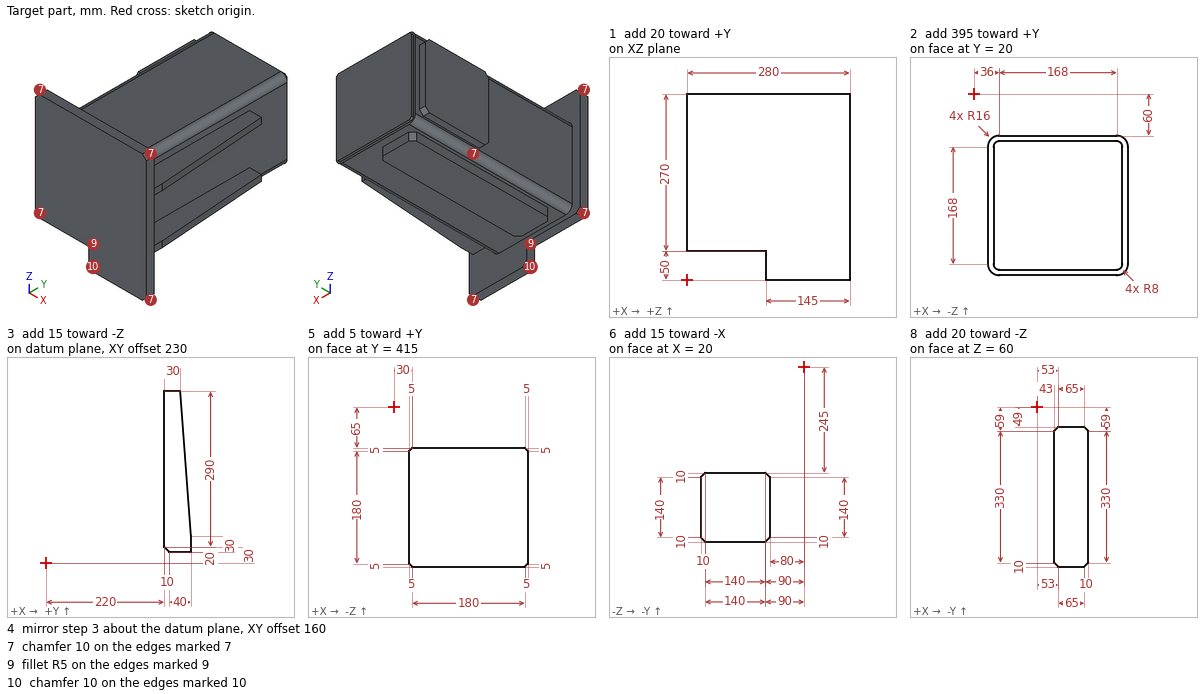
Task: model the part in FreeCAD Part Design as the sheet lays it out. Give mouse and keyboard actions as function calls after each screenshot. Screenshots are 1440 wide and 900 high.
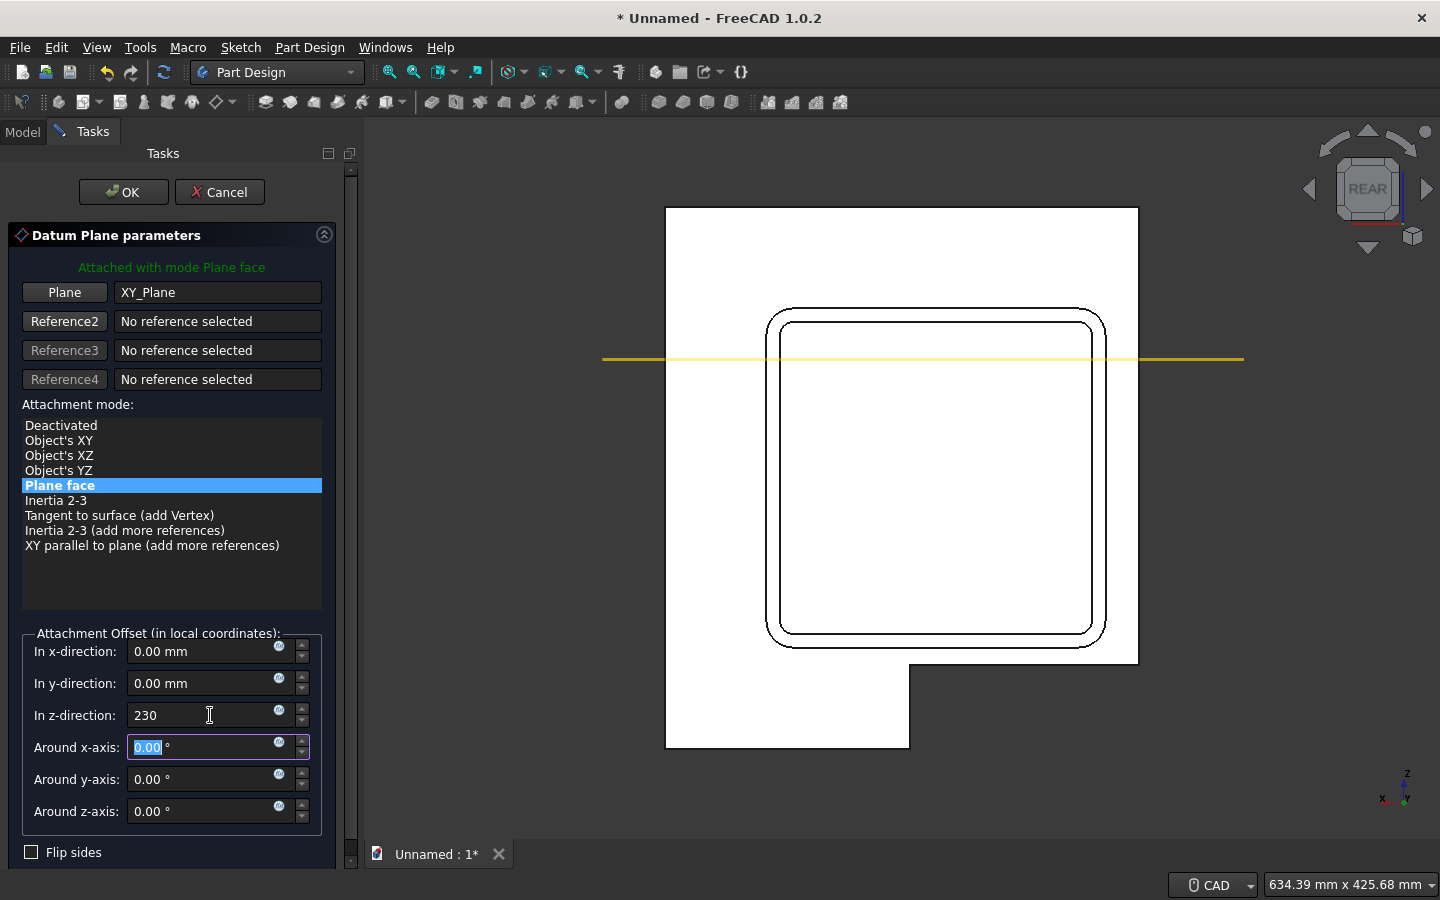
click(124, 192)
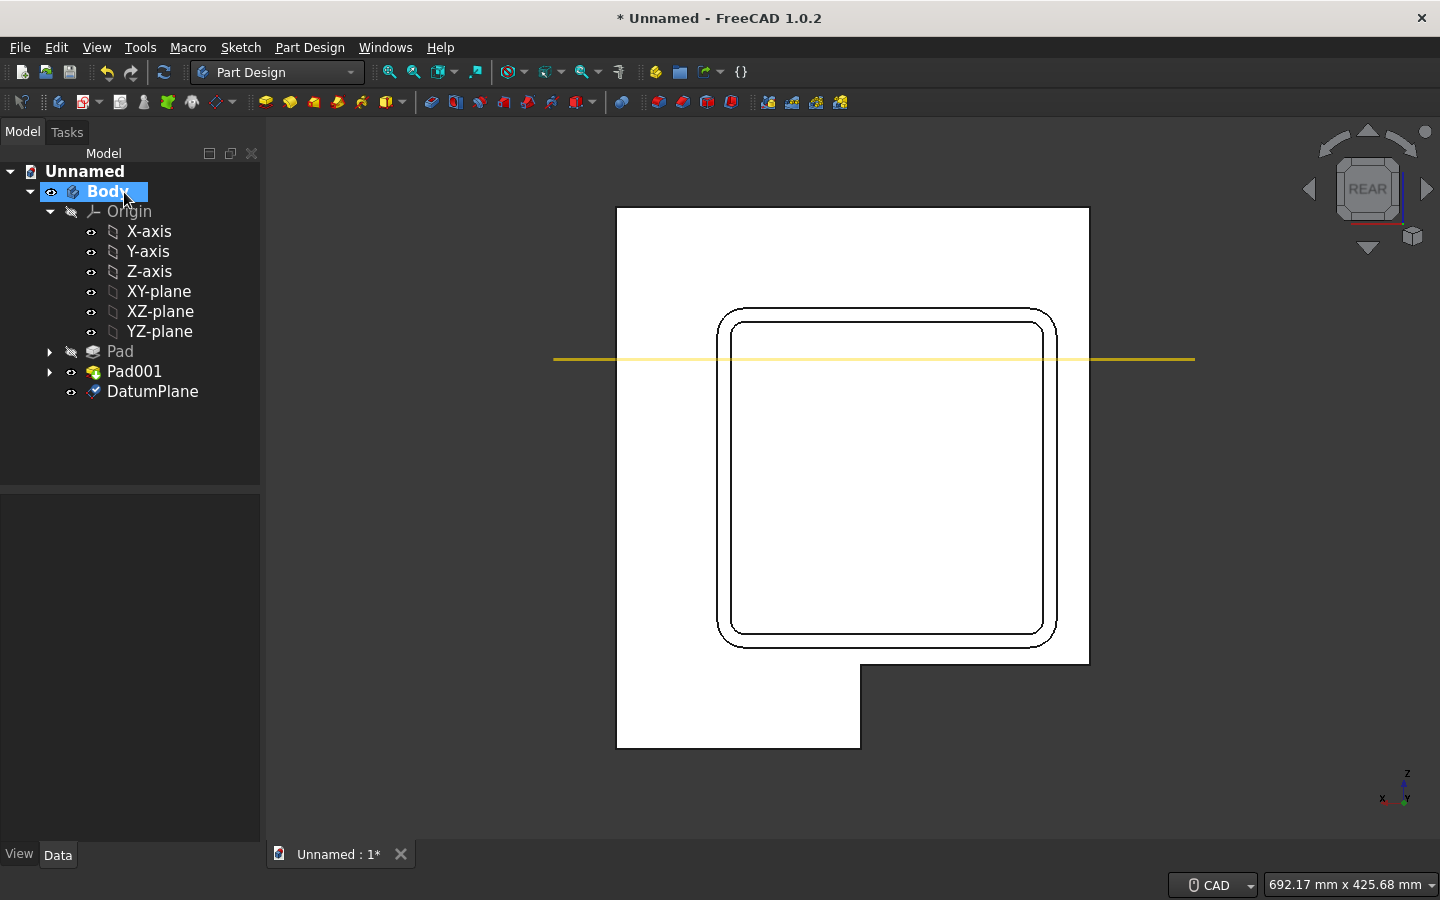
click(116, 392)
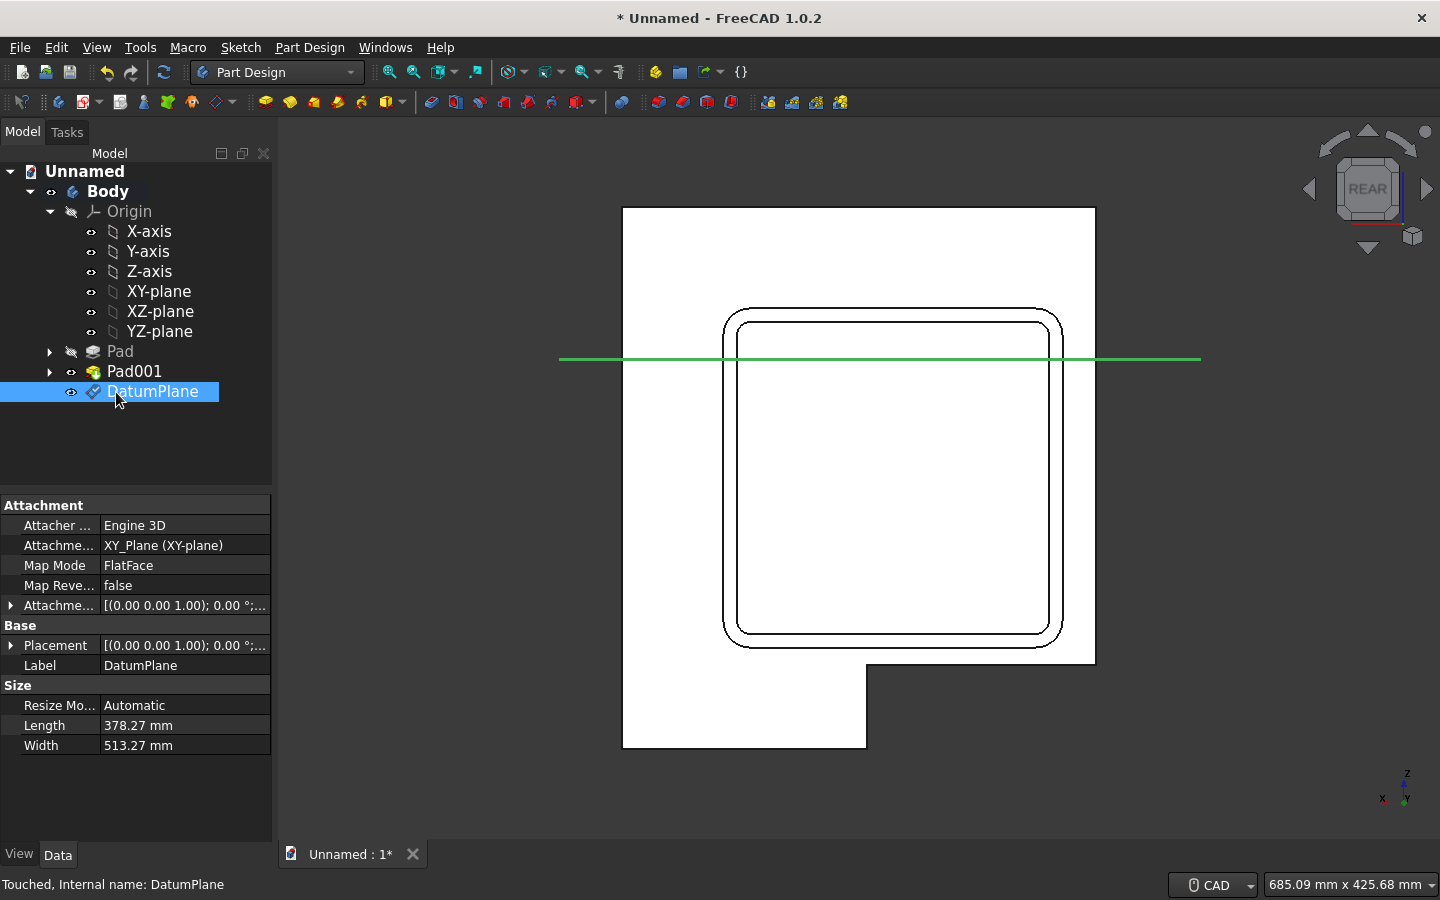
click(84, 102)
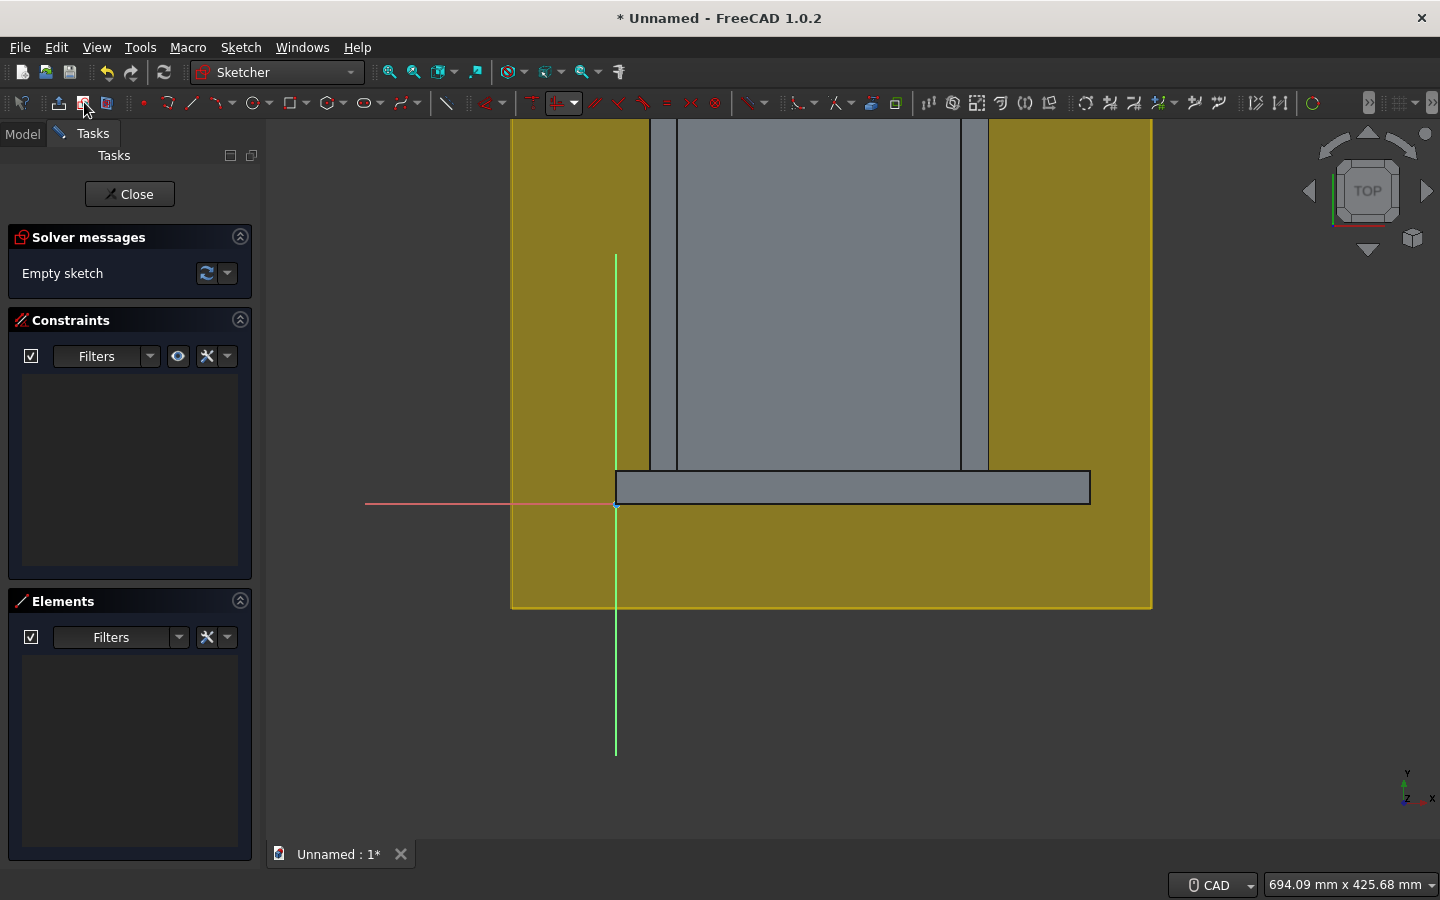
click(108, 104)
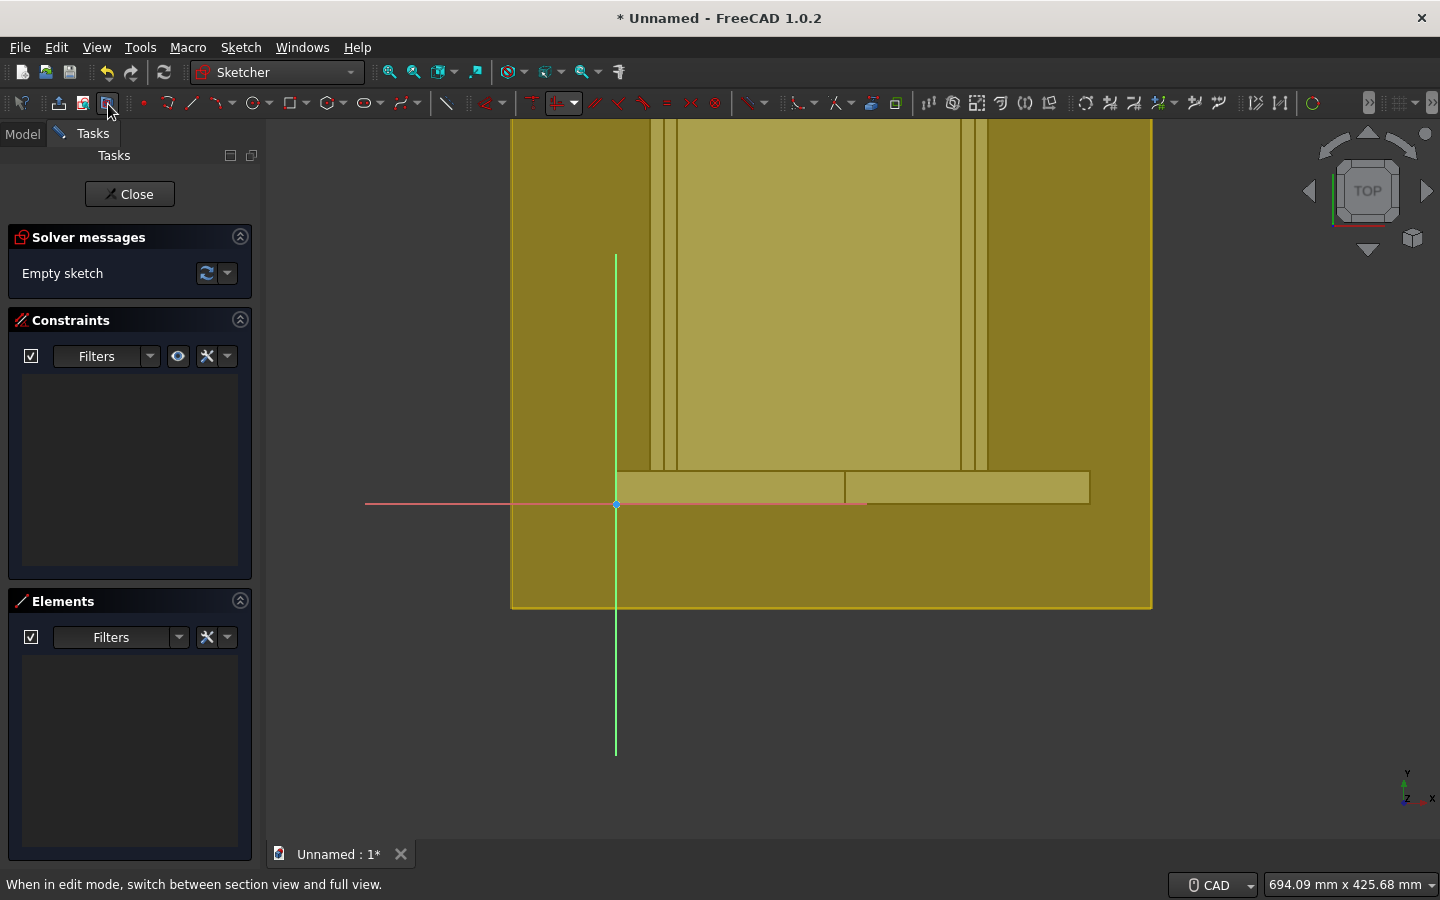
scroll(662, 811, down, 2)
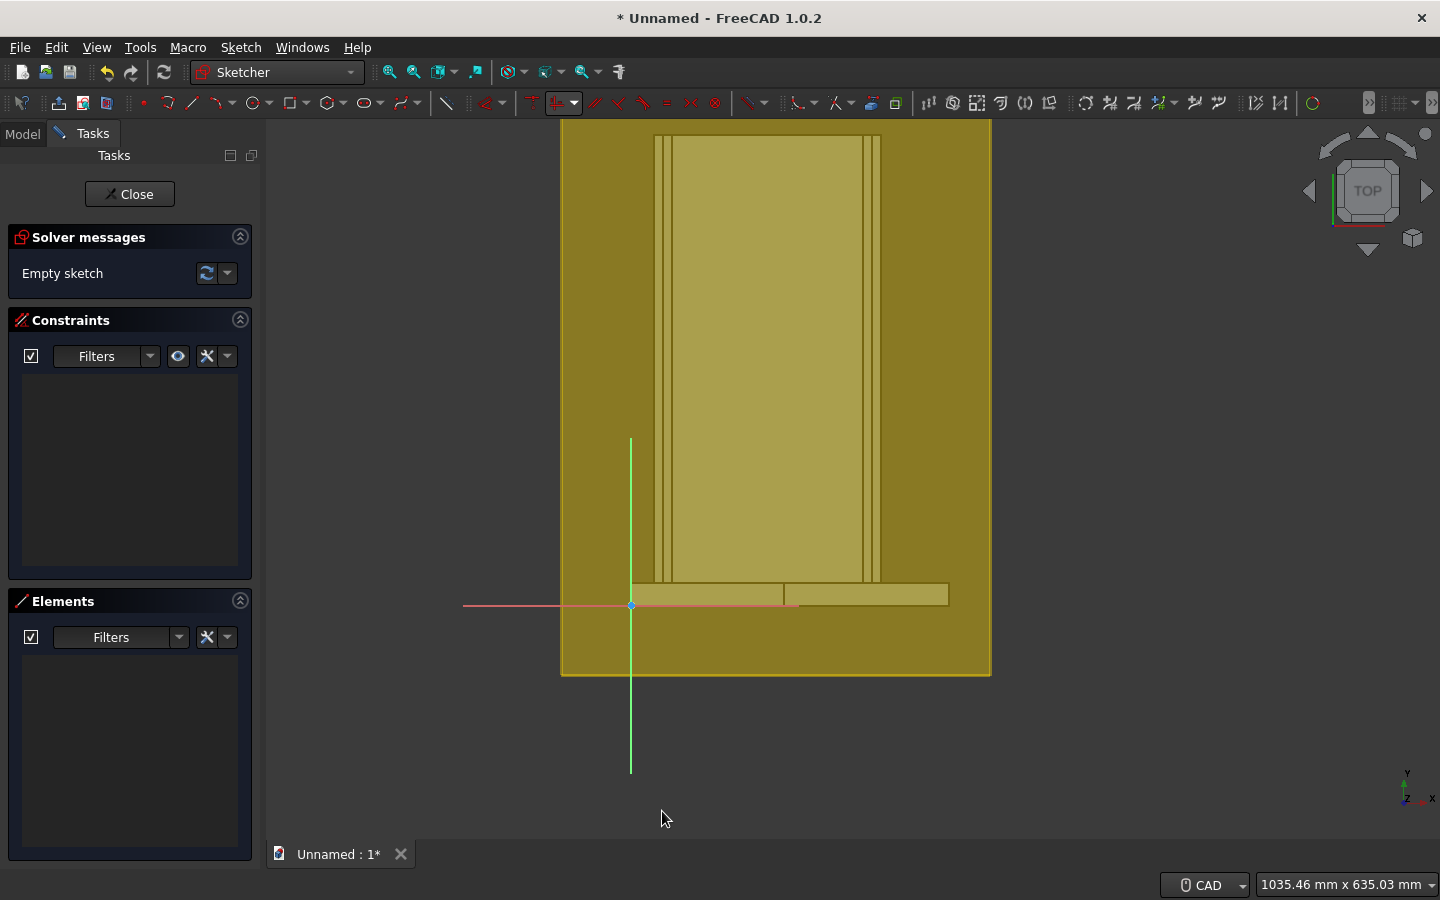
click(168, 104)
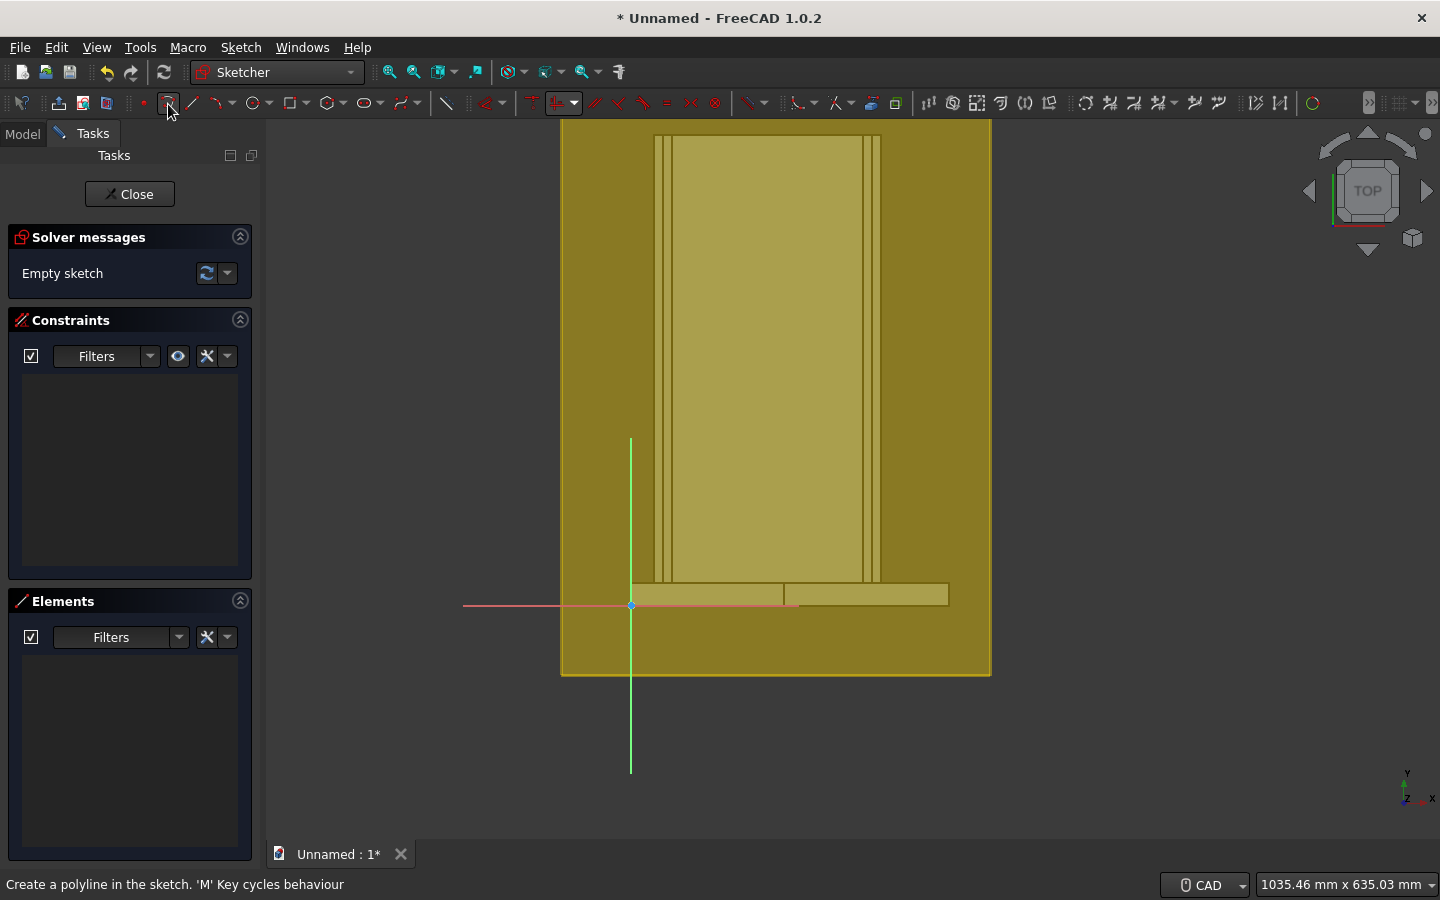
click(881, 572)
click(892, 583)
click(938, 583)
click(938, 549)
click(915, 243)
click(881, 243)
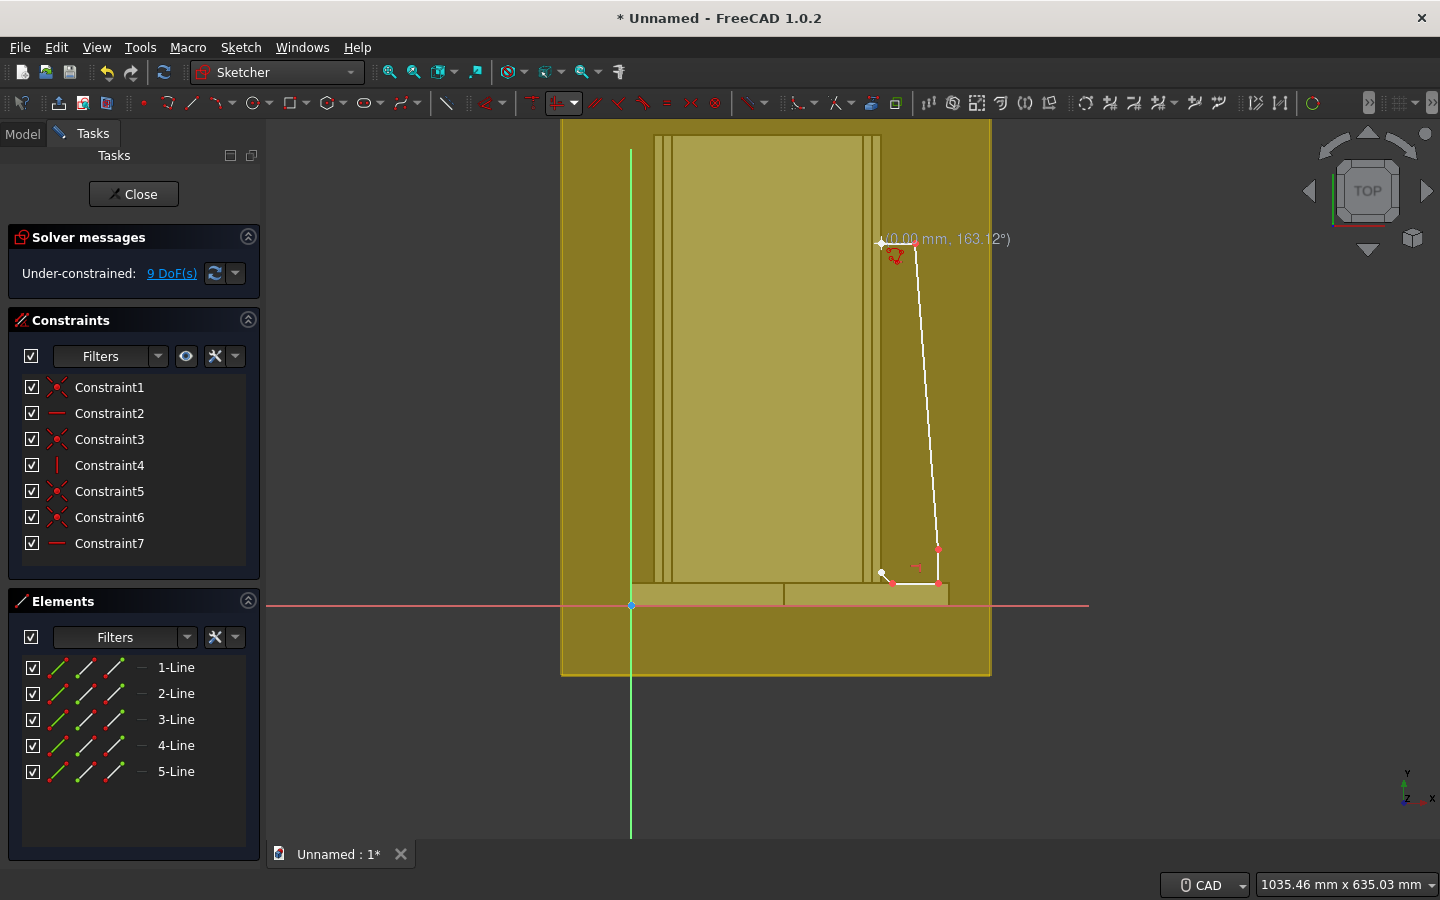
scroll(881, 572, up, 4)